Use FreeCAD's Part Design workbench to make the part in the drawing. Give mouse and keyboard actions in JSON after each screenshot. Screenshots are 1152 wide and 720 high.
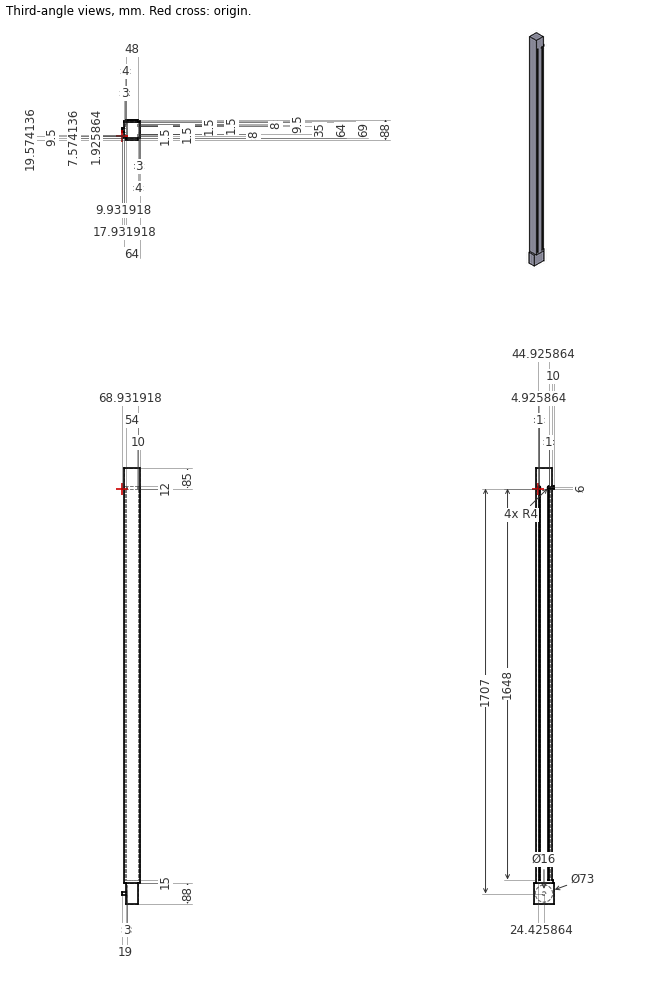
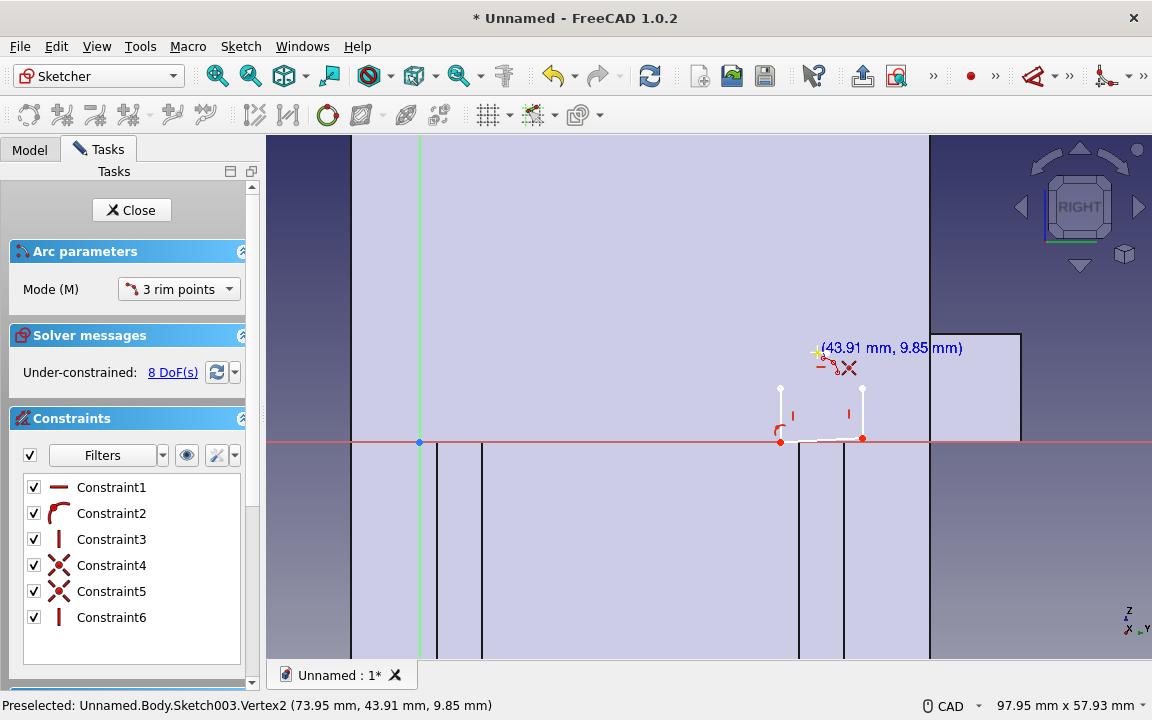
{"action": "left_click", "coordinate": [781, 389]}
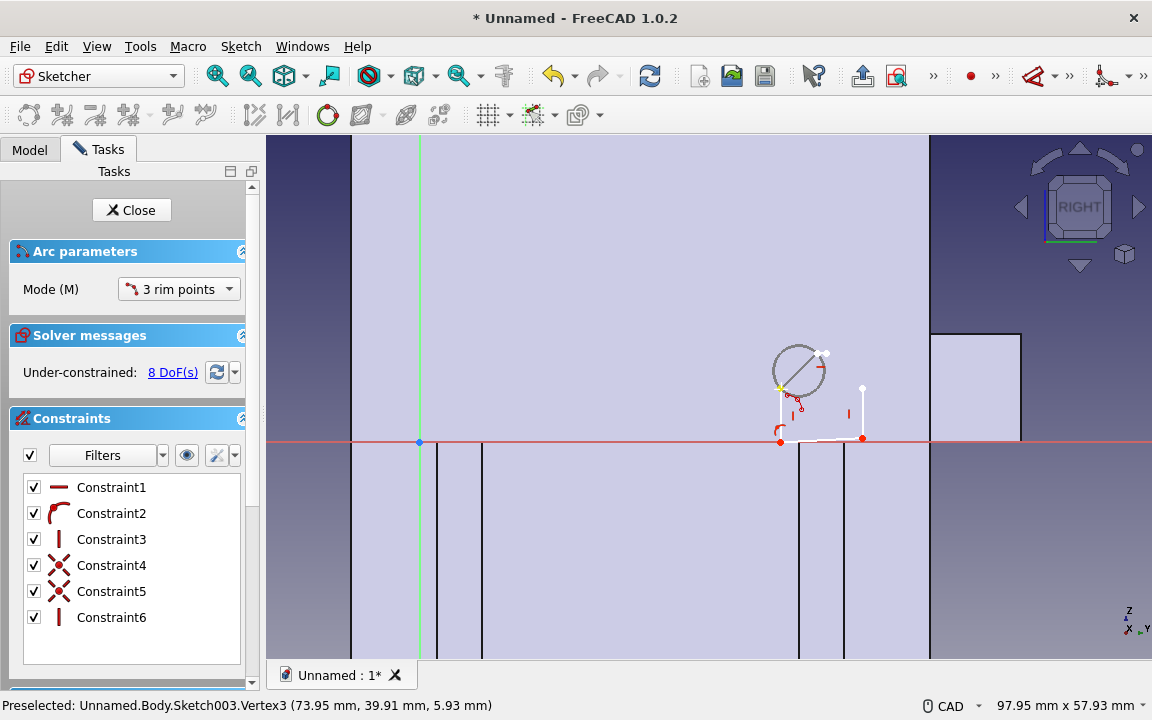
{"action": "scroll", "coordinate": [792, 363], "scroll_direction": "up", "scroll_amount": 3}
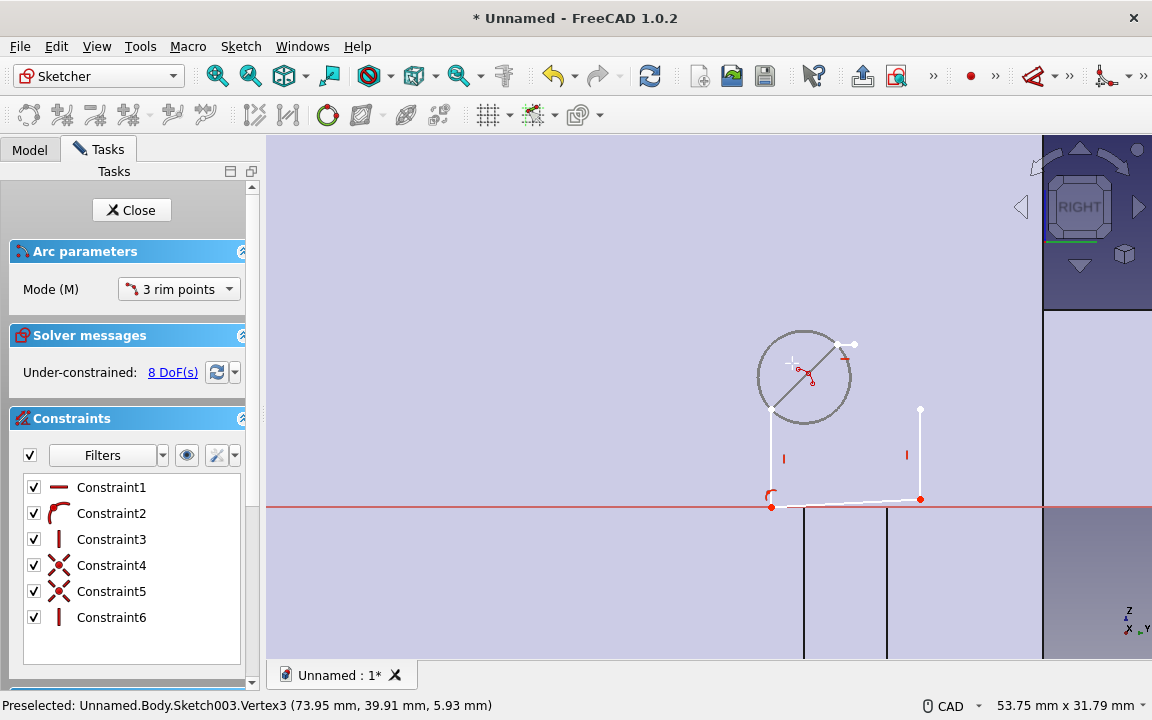
{"action": "left_click", "coordinate": [791, 362]}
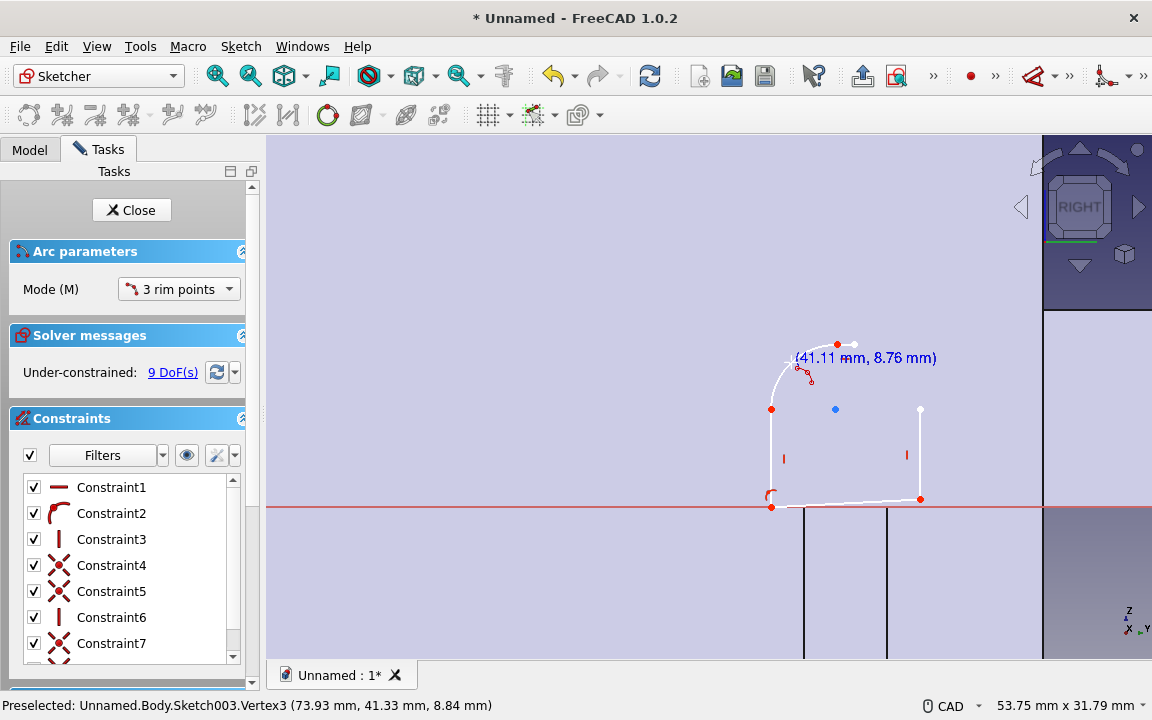
{"action": "left_click", "coordinate": [920, 409]}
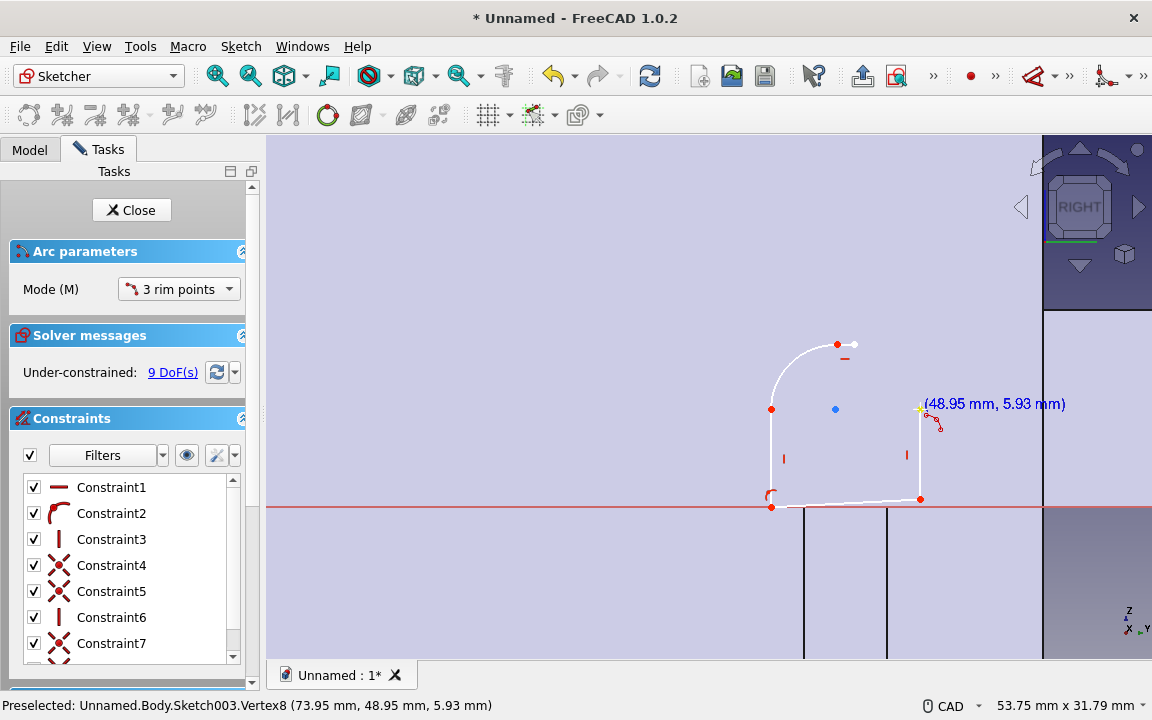
{"action": "scroll", "coordinate": [854, 342], "scroll_direction": "up", "scroll_amount": 4}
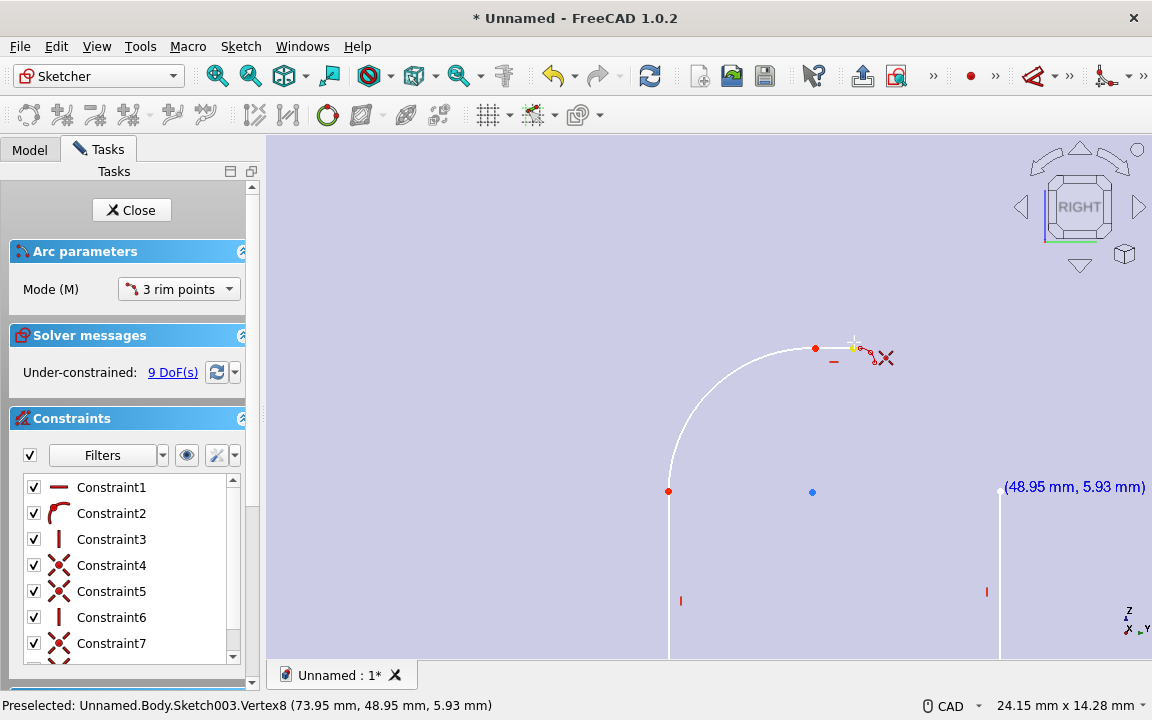
{"action": "left_click", "coordinate": [853, 348]}
{"action": "left_click", "coordinate": [957, 386]}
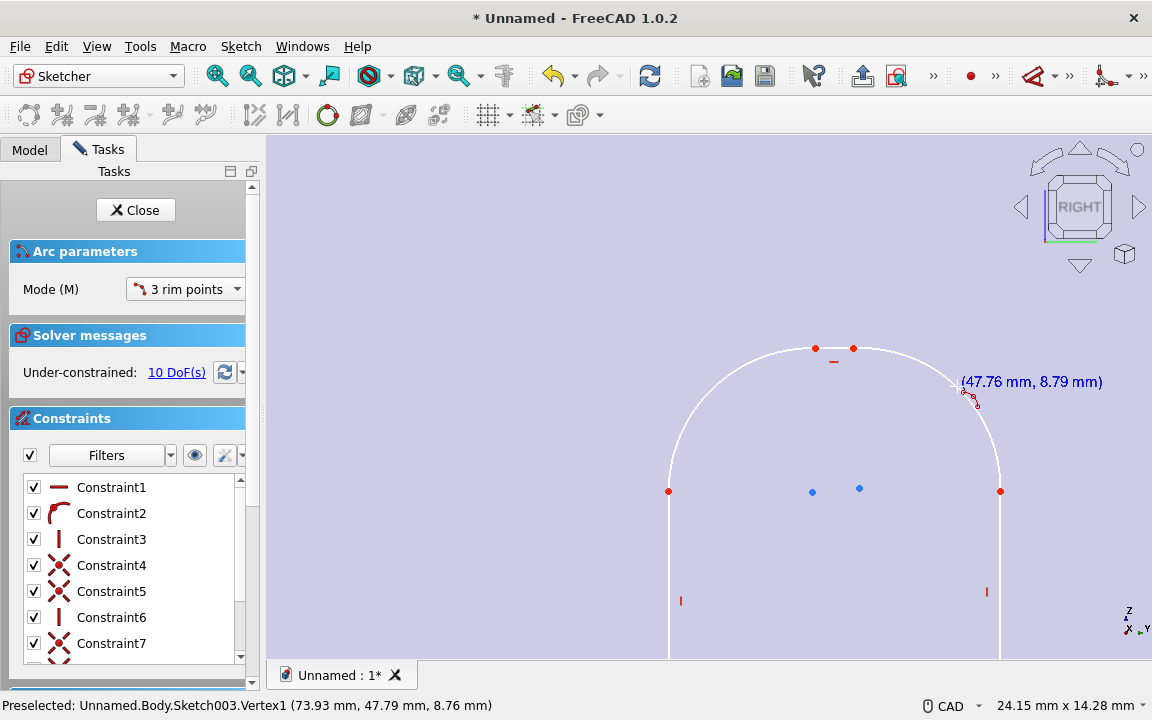
{"action": "key", "text": "g l"}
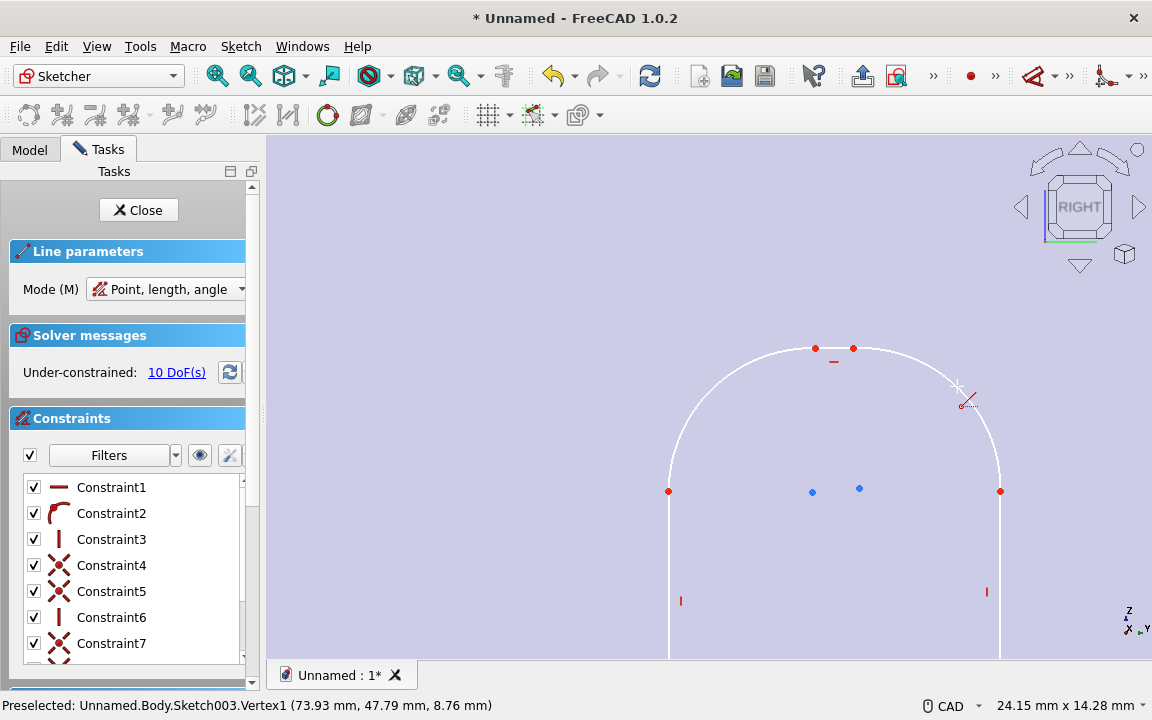
{"action": "scroll", "coordinate": [817, 355], "scroll_direction": "down", "scroll_amount": 7}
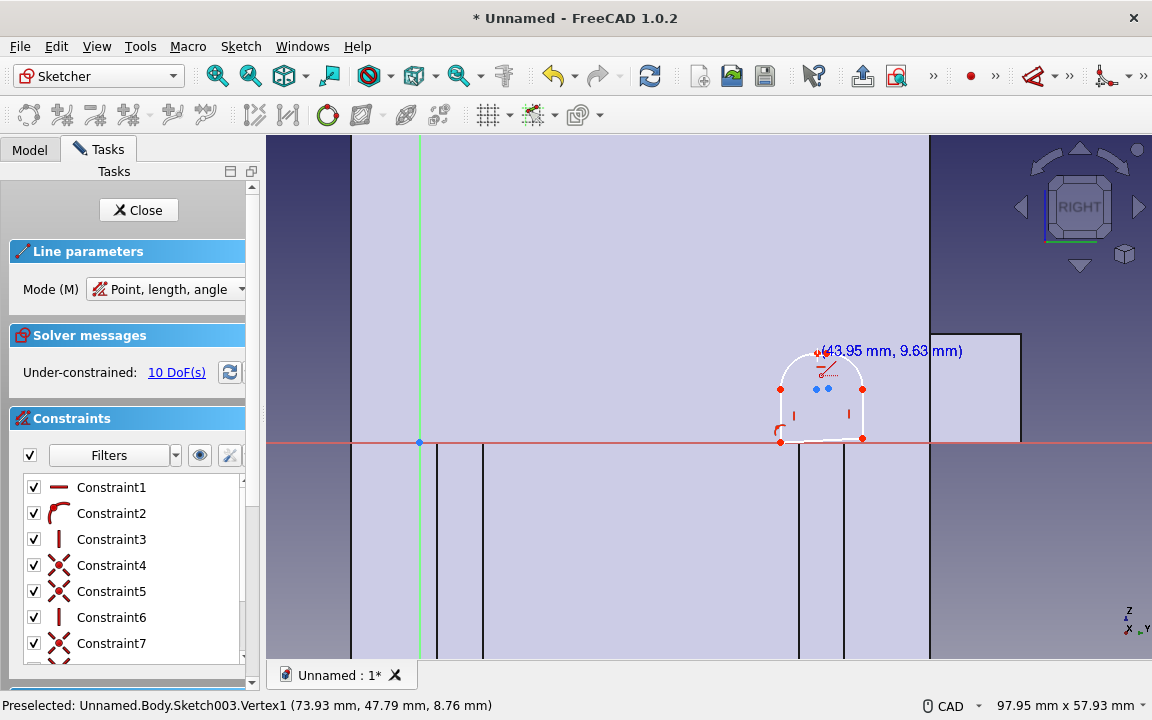
{"action": "left_click", "coordinate": [464, 352]}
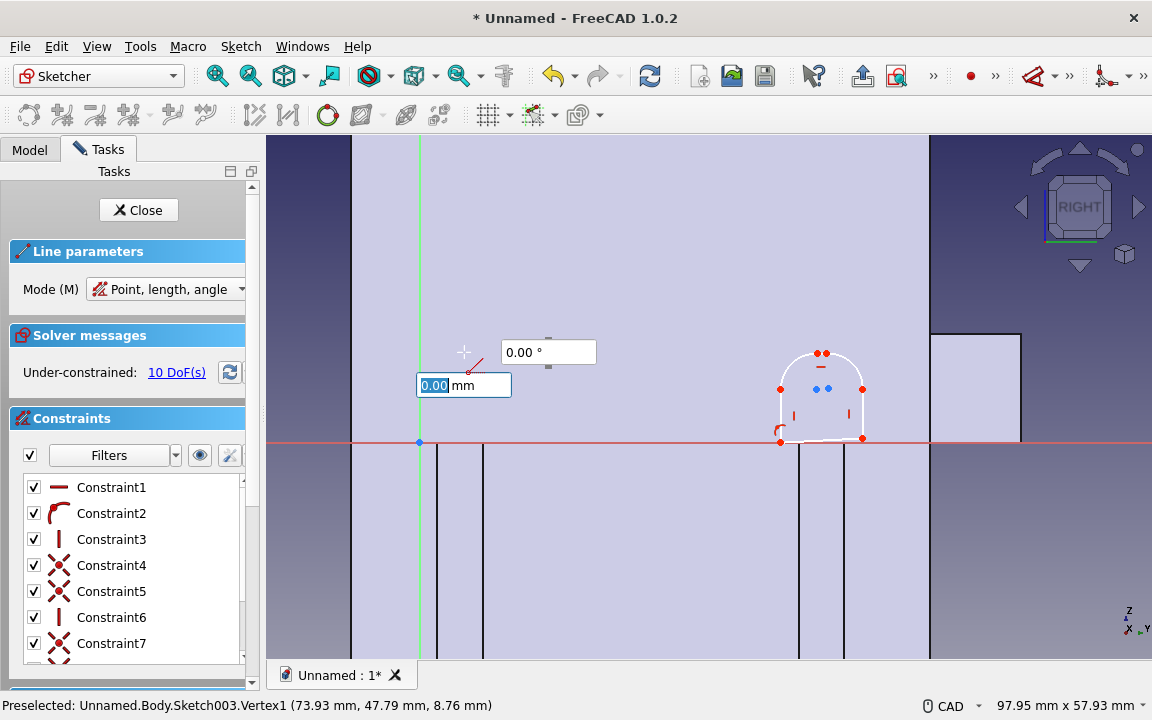
{"action": "scroll", "coordinate": [455, 352], "scroll_direction": "up", "scroll_amount": 3}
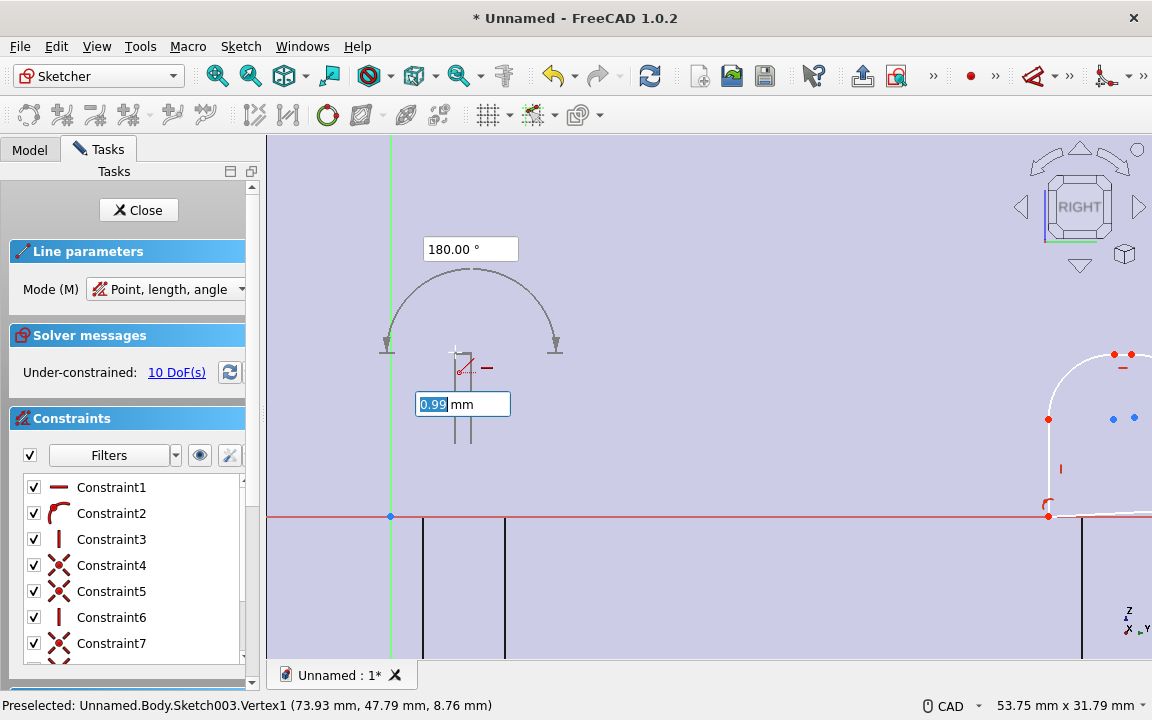
{"action": "left_click", "coordinate": [456, 352]}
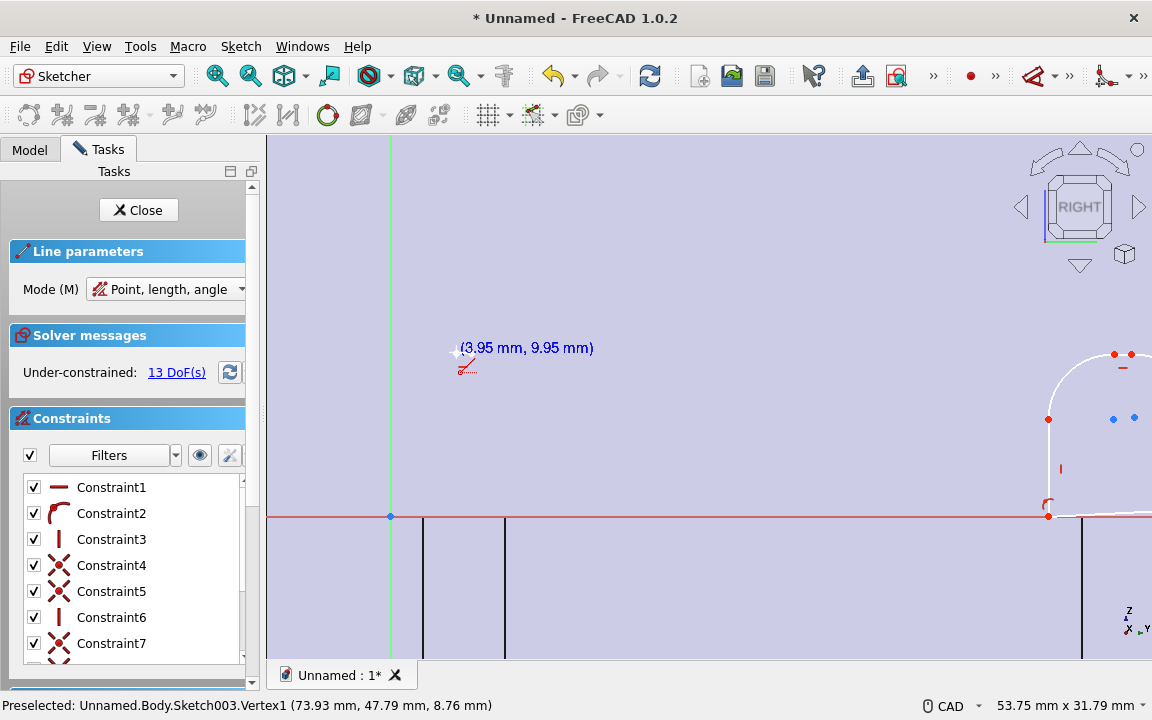
{"action": "key", "text": "g m"}